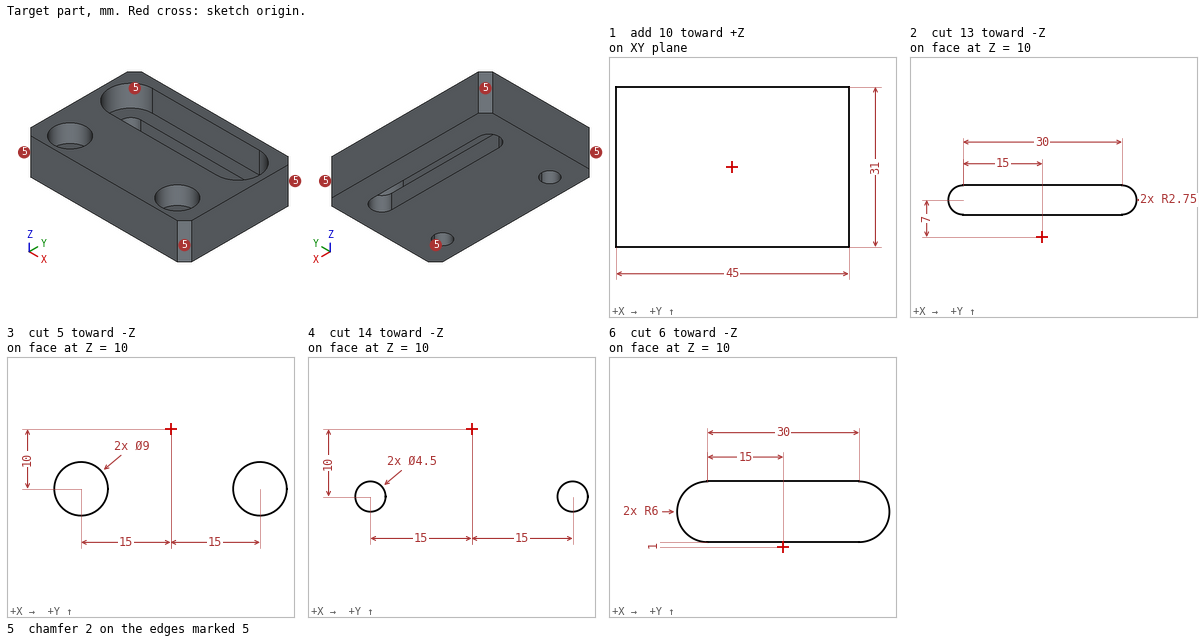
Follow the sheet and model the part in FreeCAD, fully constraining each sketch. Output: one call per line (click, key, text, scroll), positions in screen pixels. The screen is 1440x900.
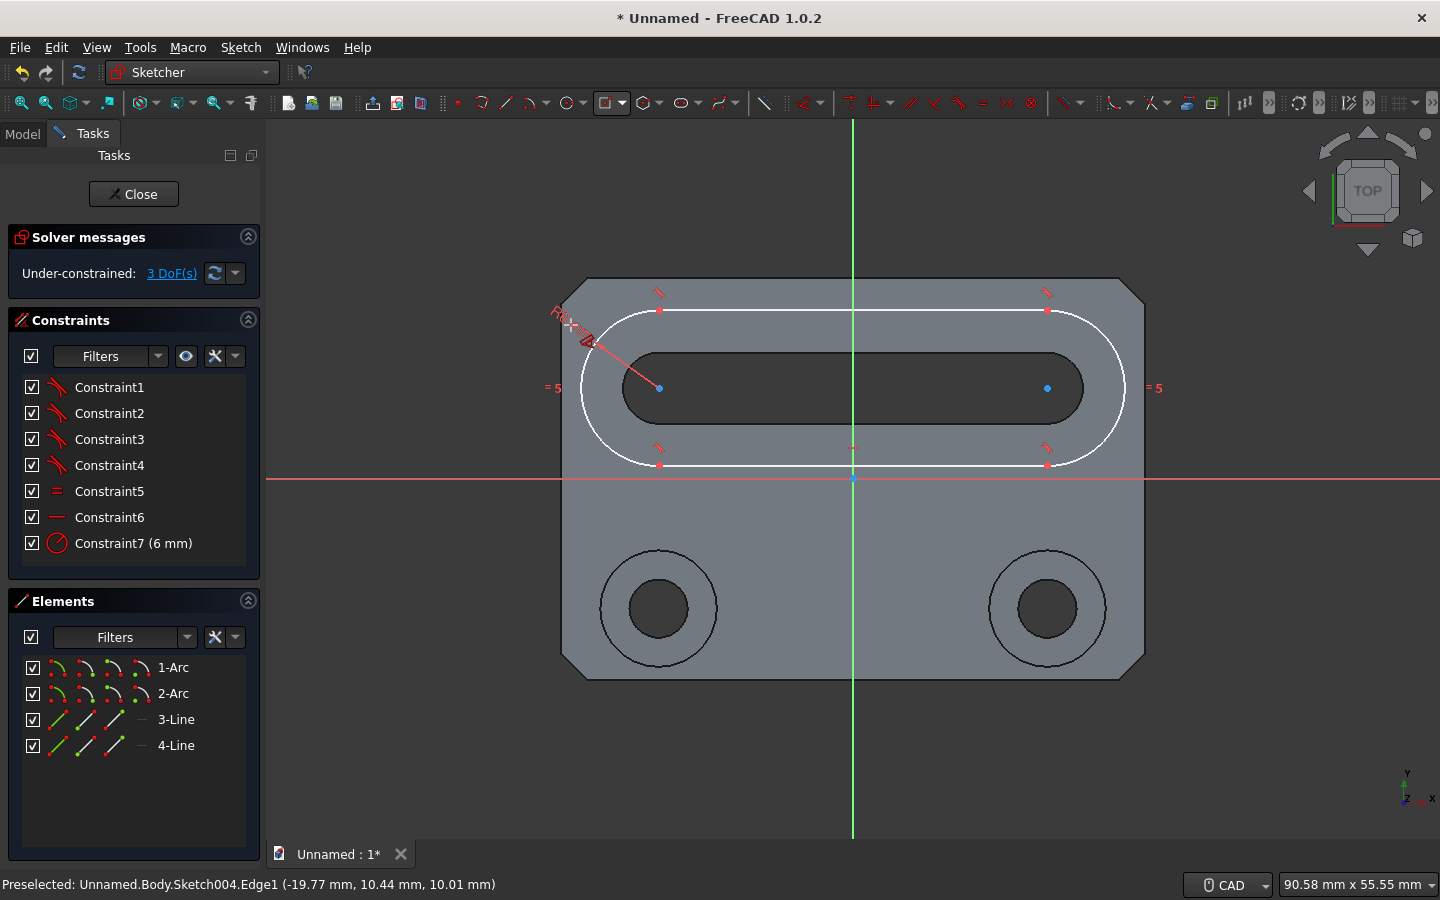
click(775, 310)
click(764, 276)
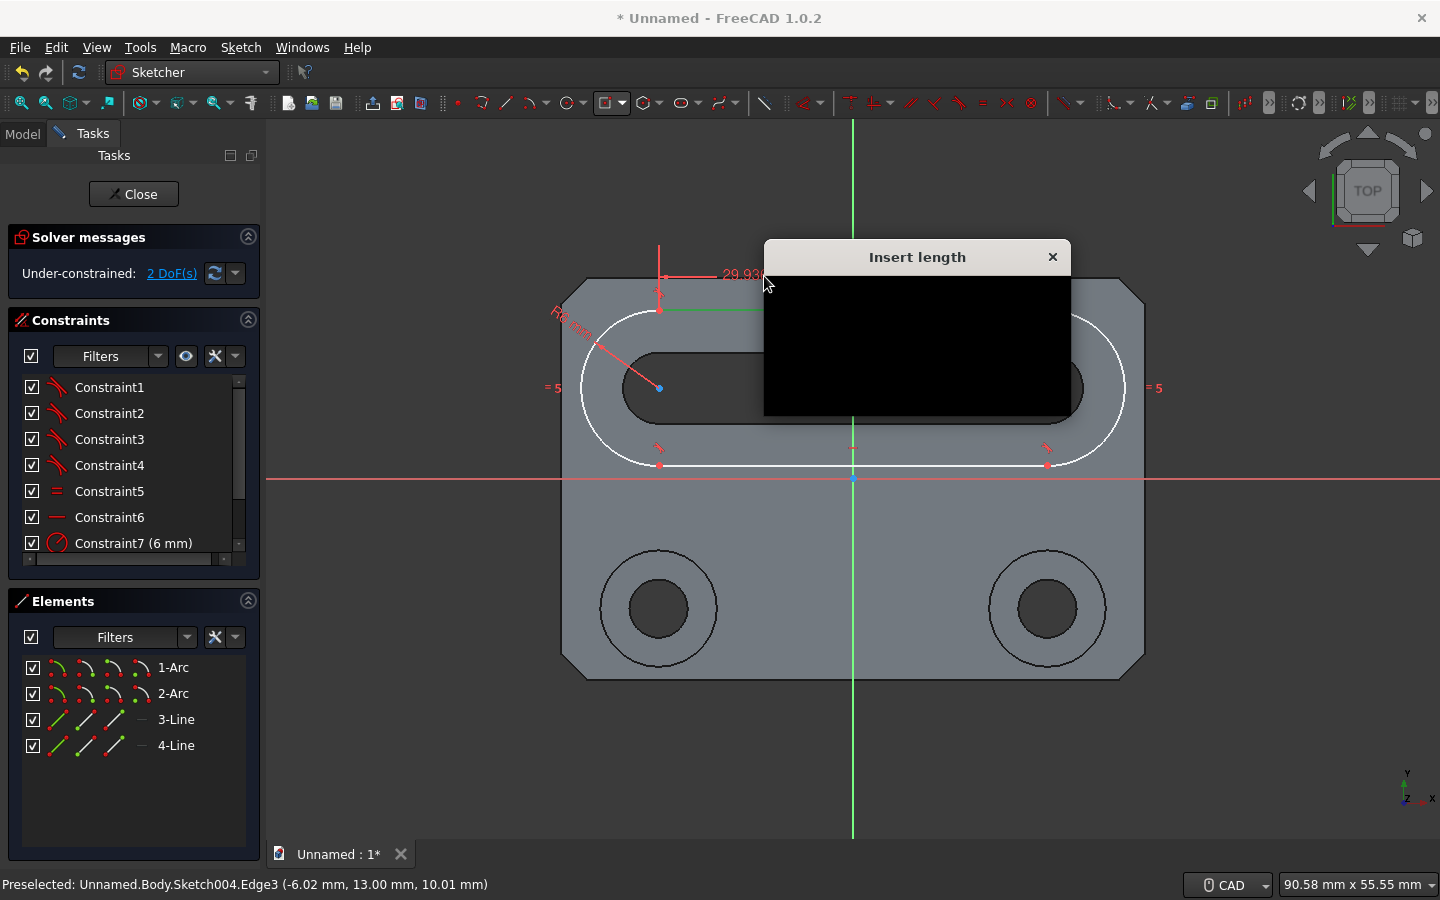
text(30)
key(Return)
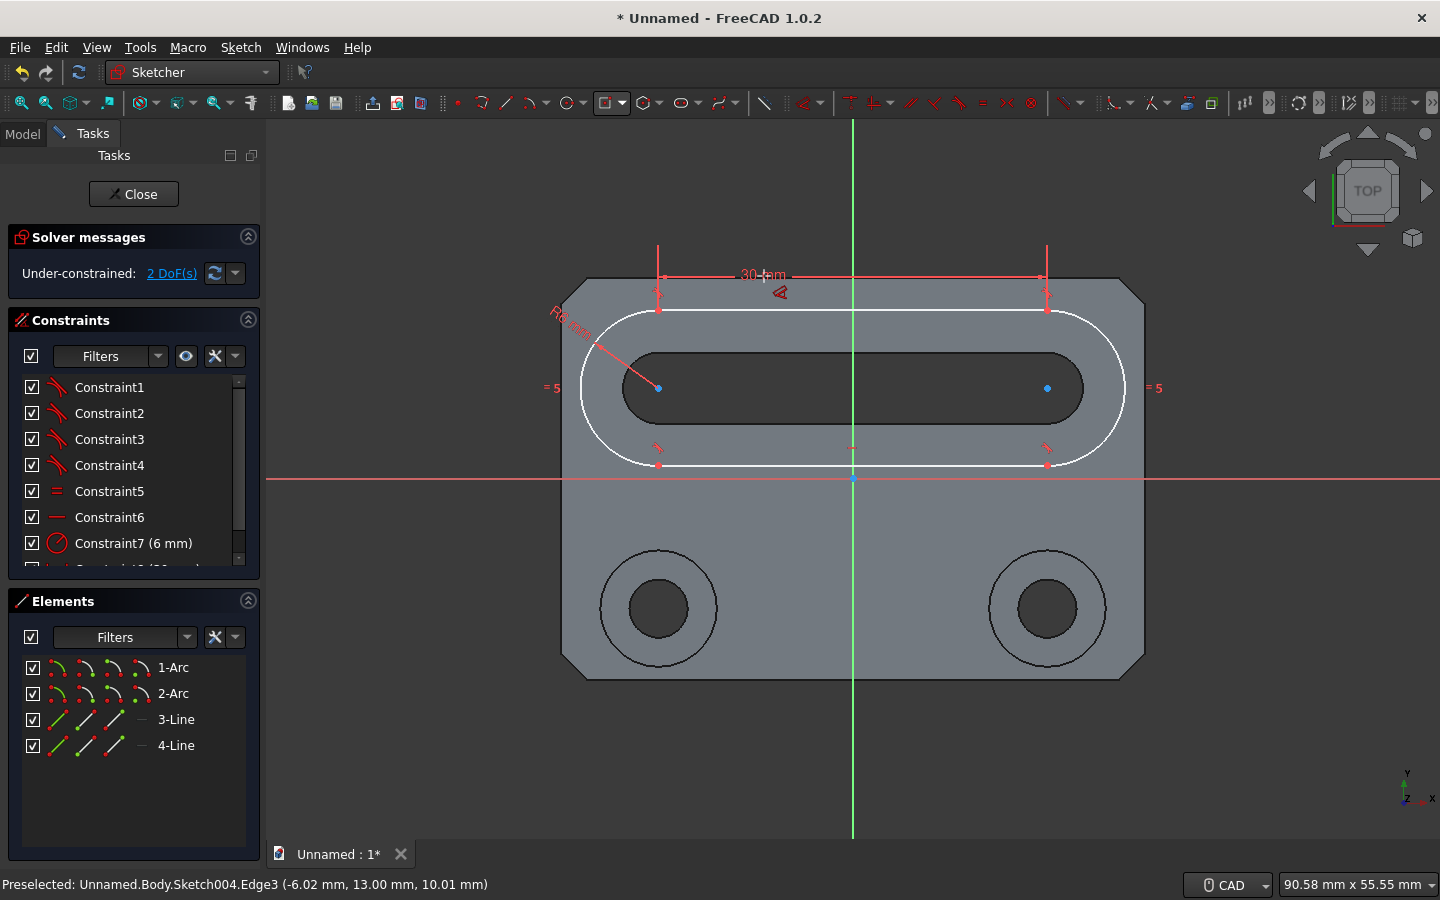
scroll(658, 466, up, 6)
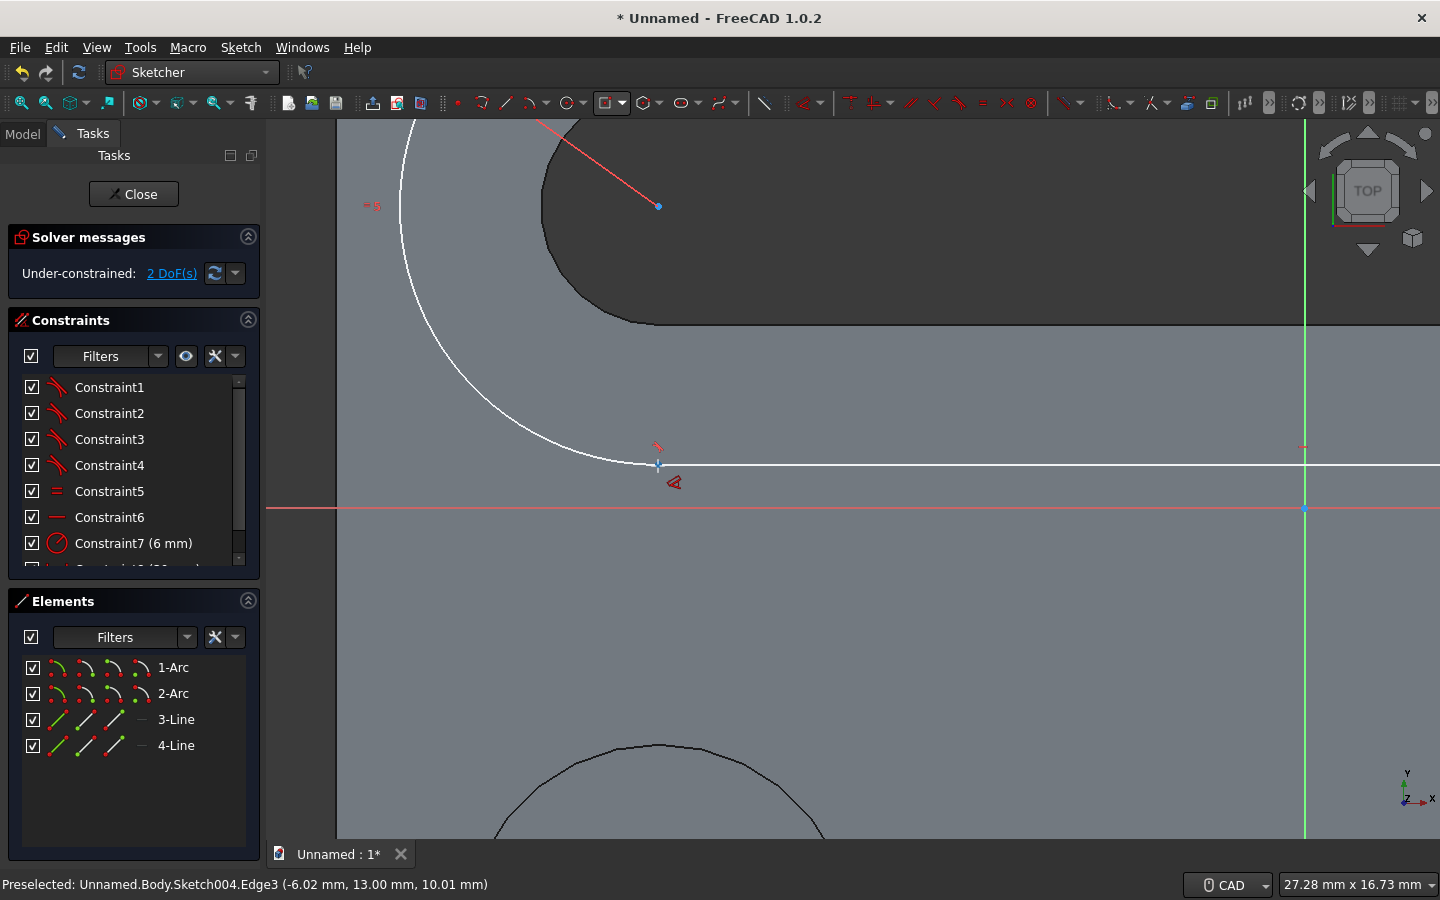
click(658, 465)
click(624, 486)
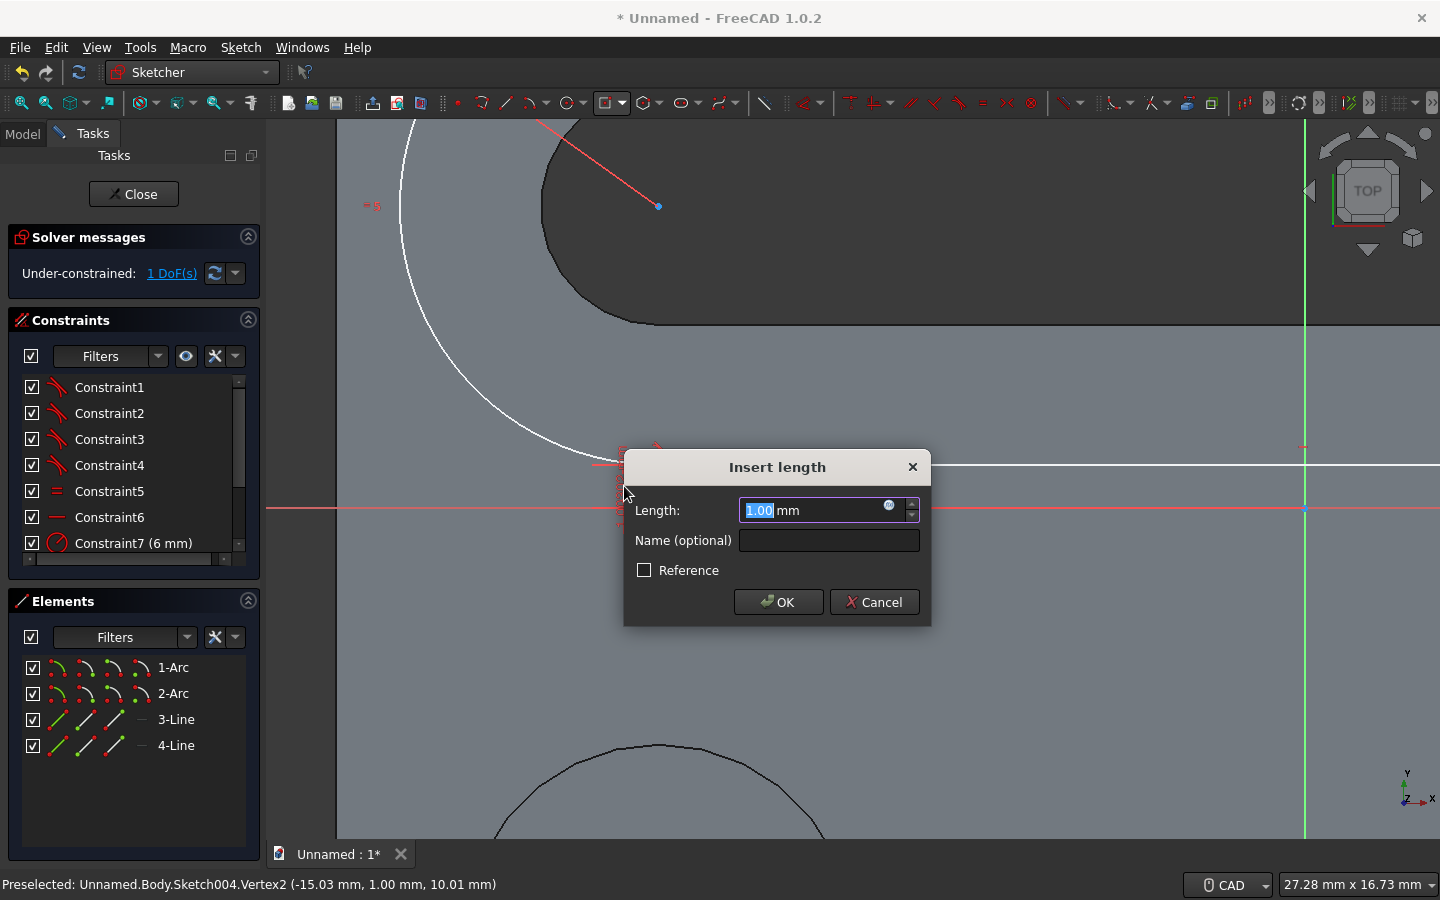
text(1)
key(Return)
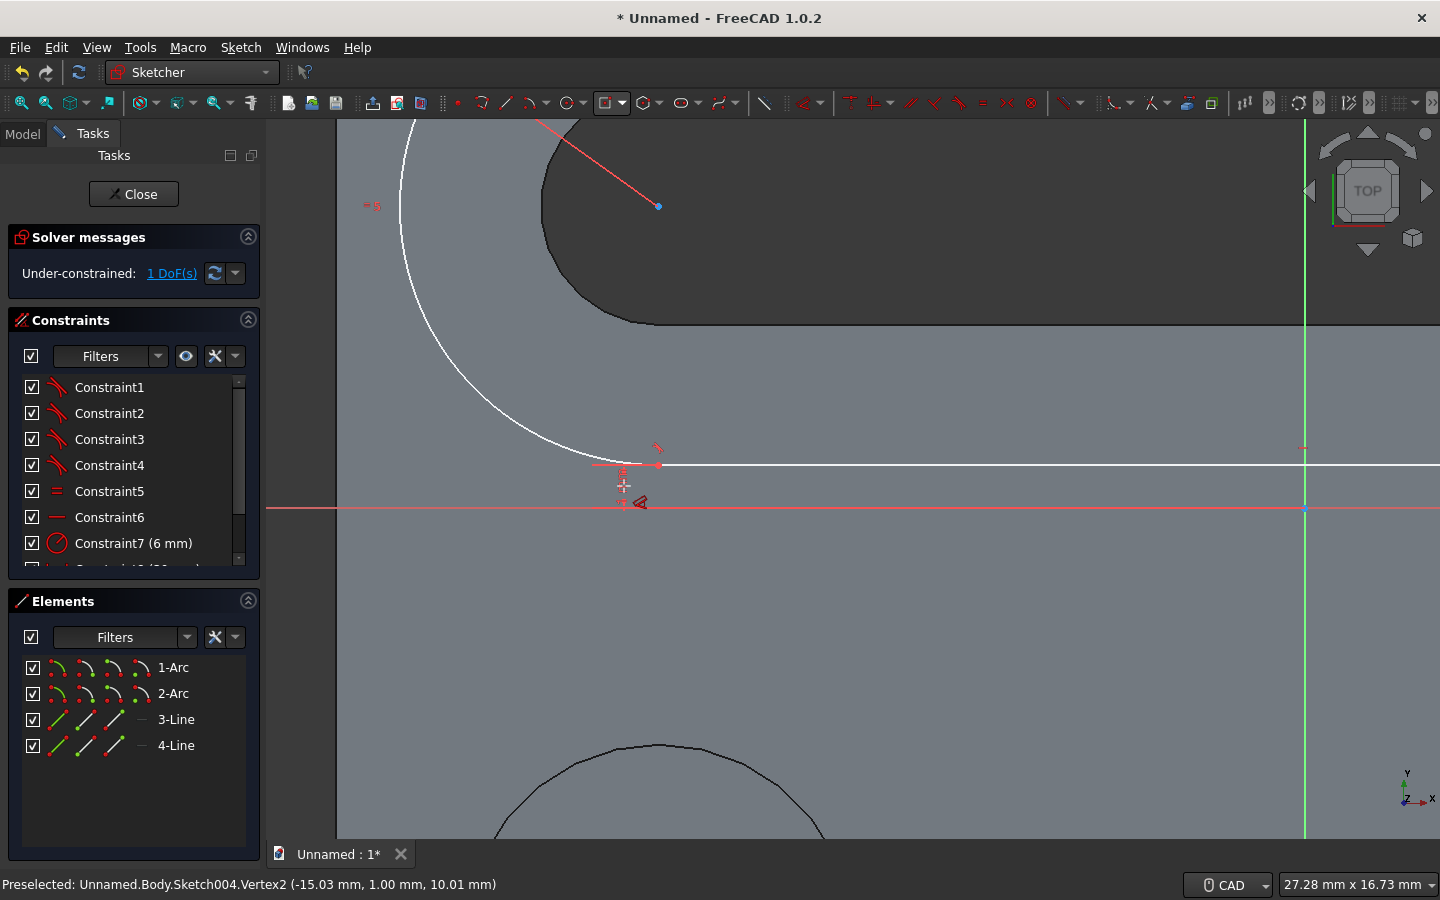
scroll(482, 625, down, 5)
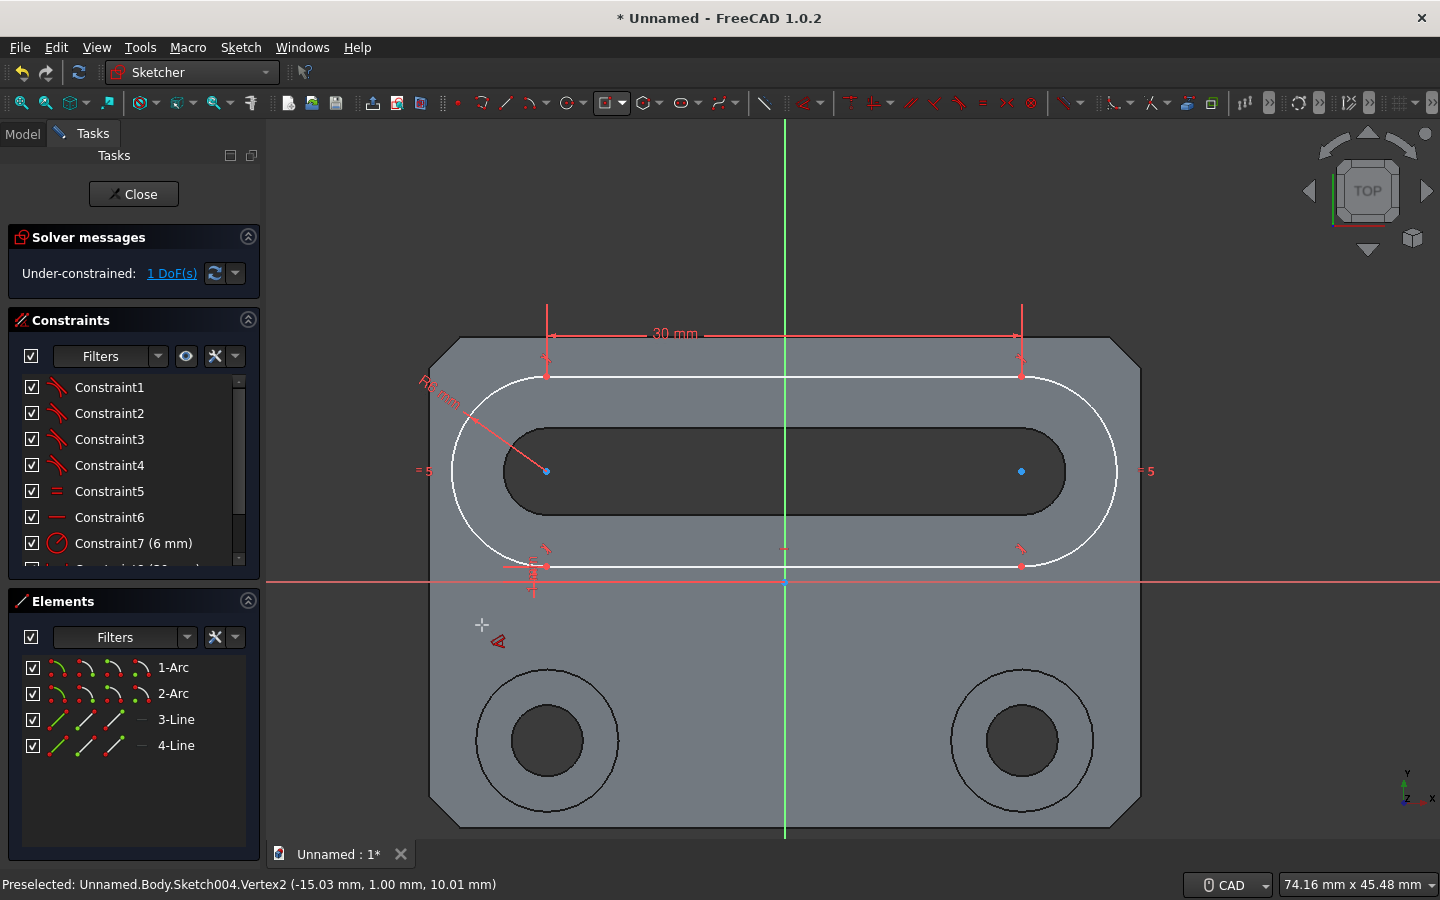
click(547, 377)
click(666, 616)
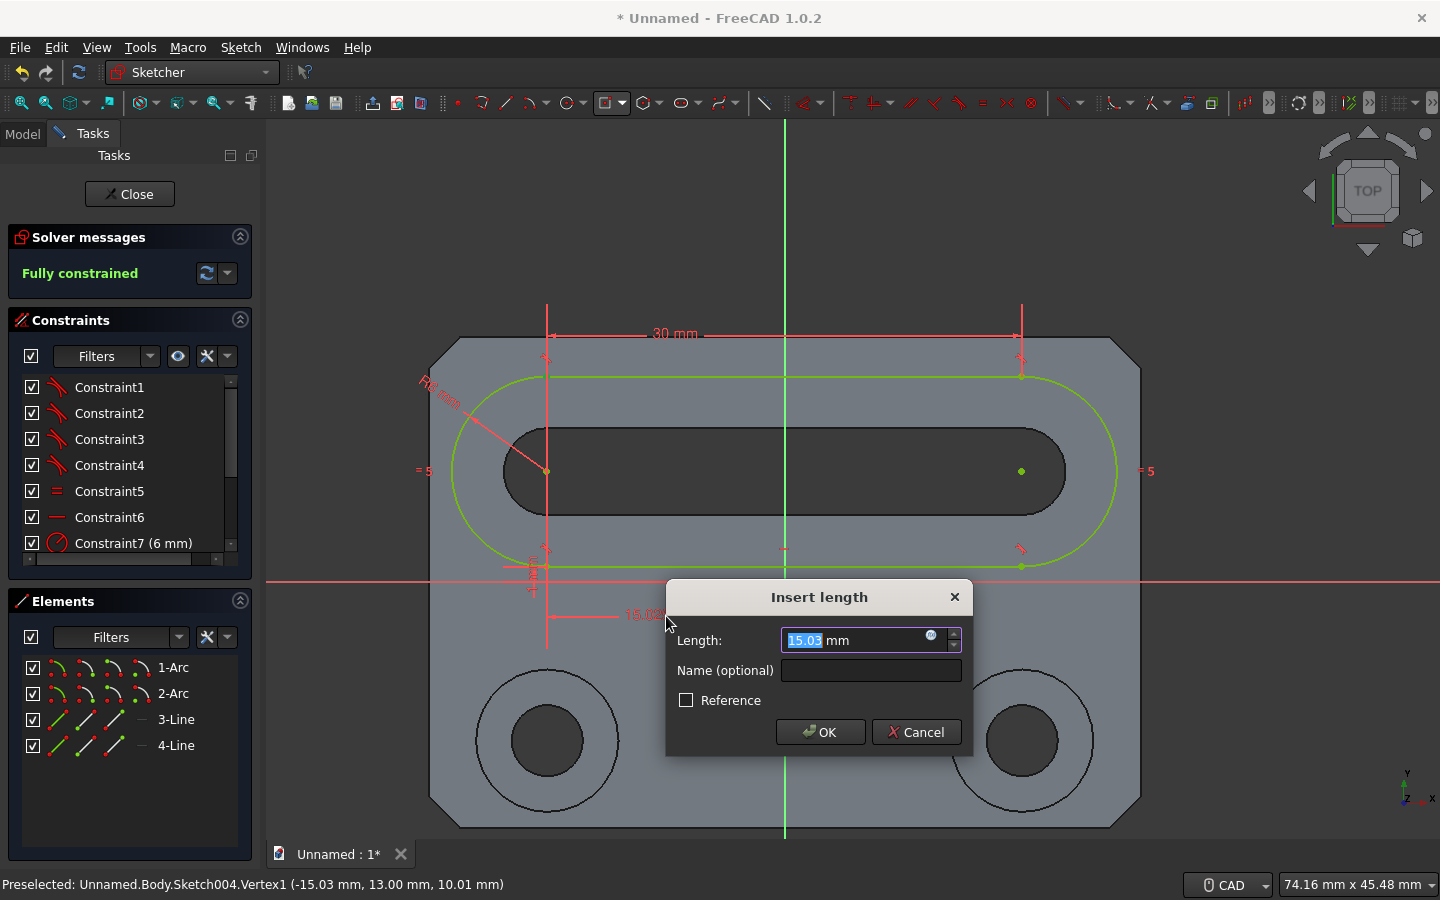
text(15)
key(Return)
key(Escape)